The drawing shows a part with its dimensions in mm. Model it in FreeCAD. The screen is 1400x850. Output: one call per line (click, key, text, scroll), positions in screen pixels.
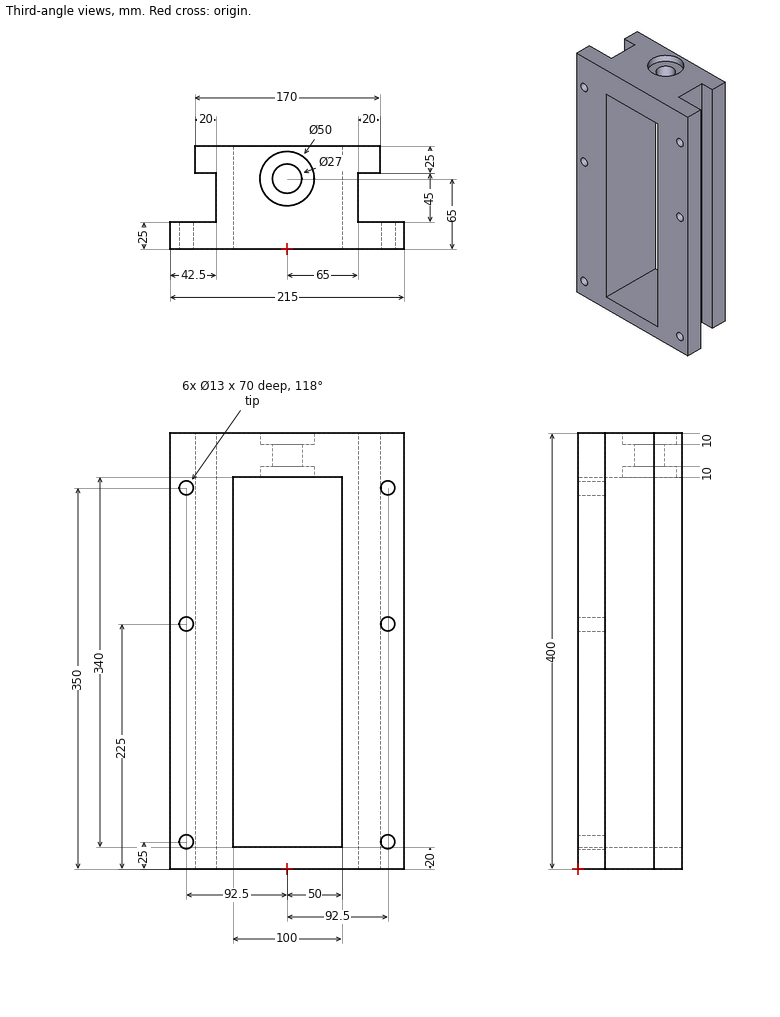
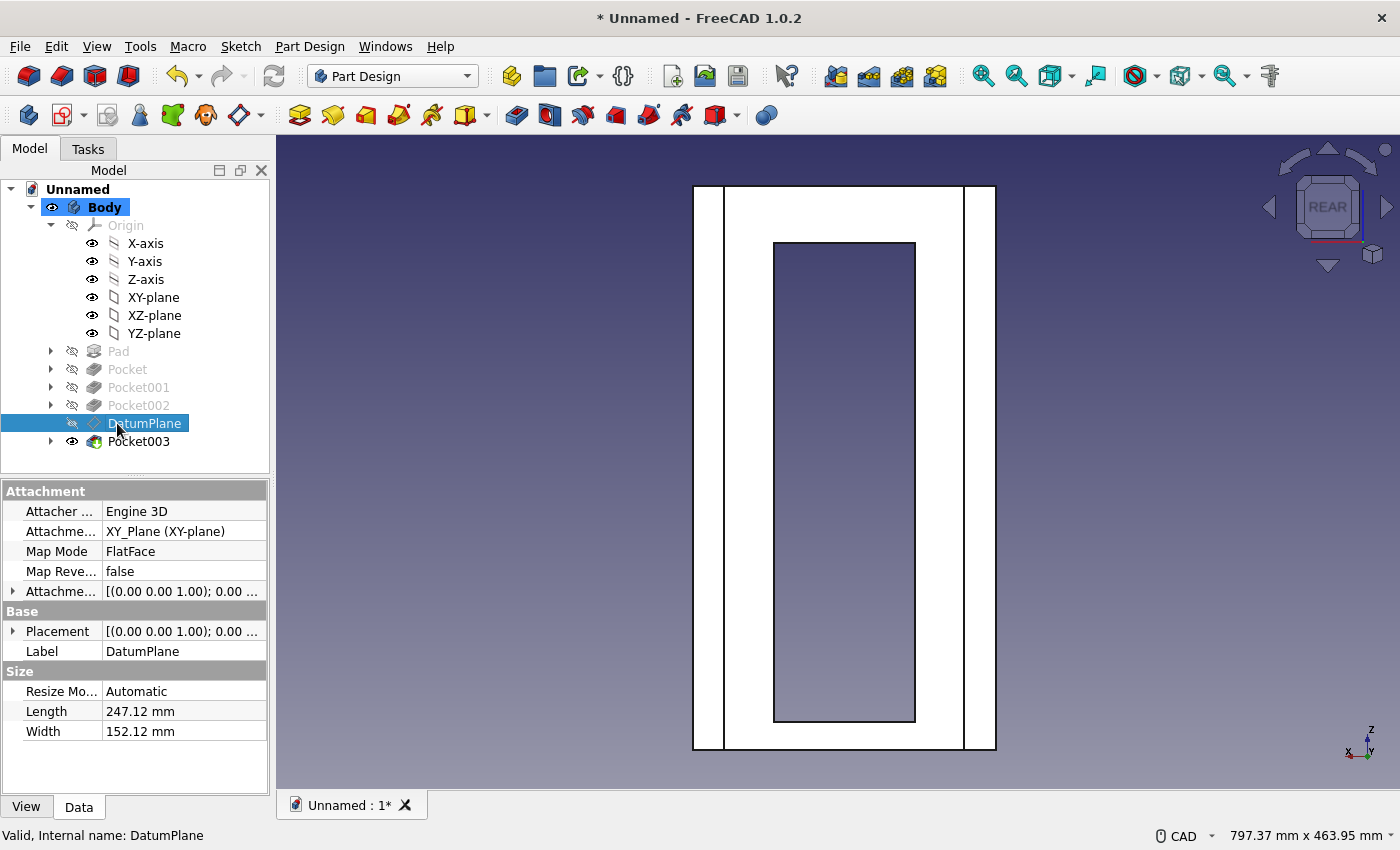
click(714, 226)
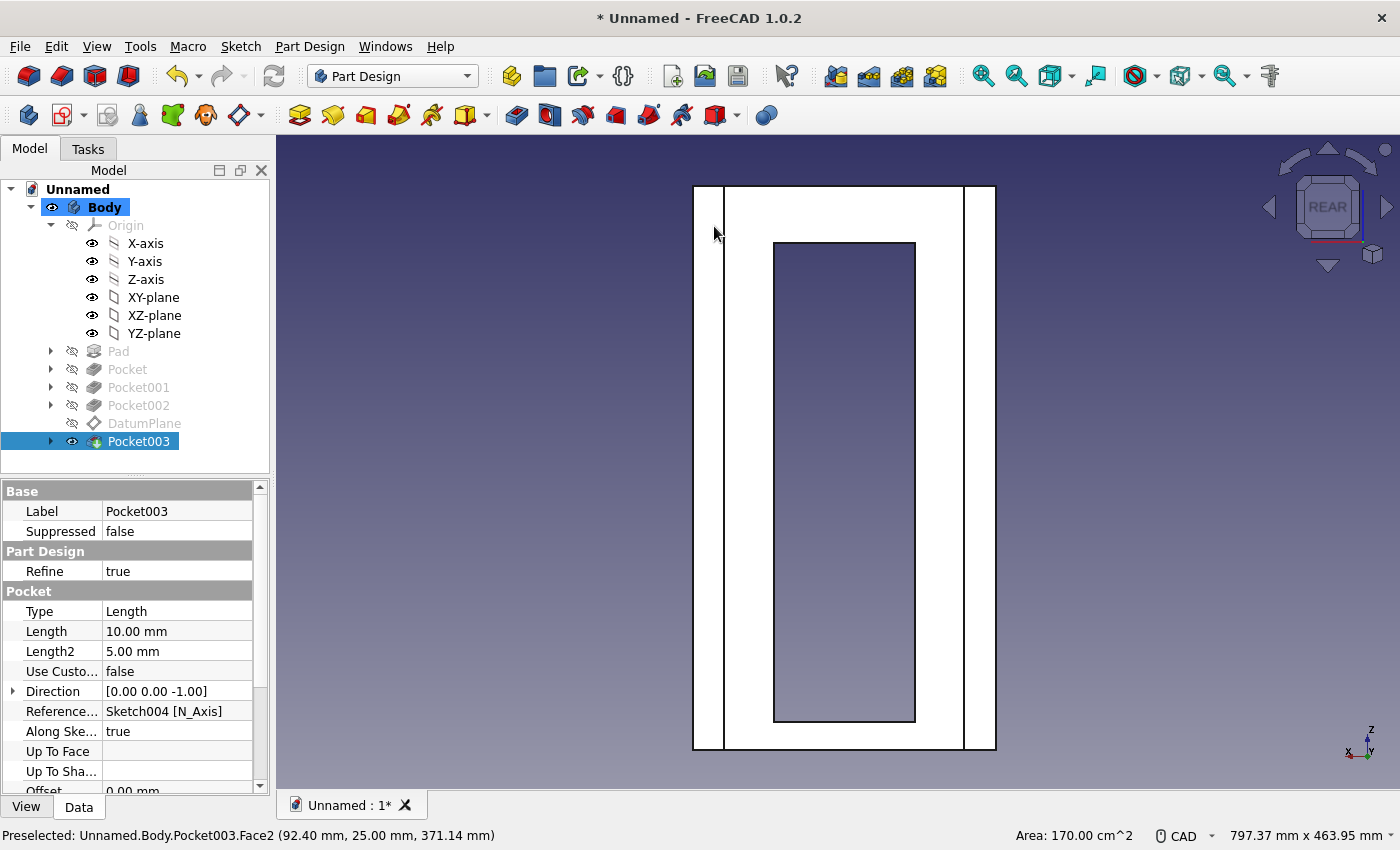
click(62, 116)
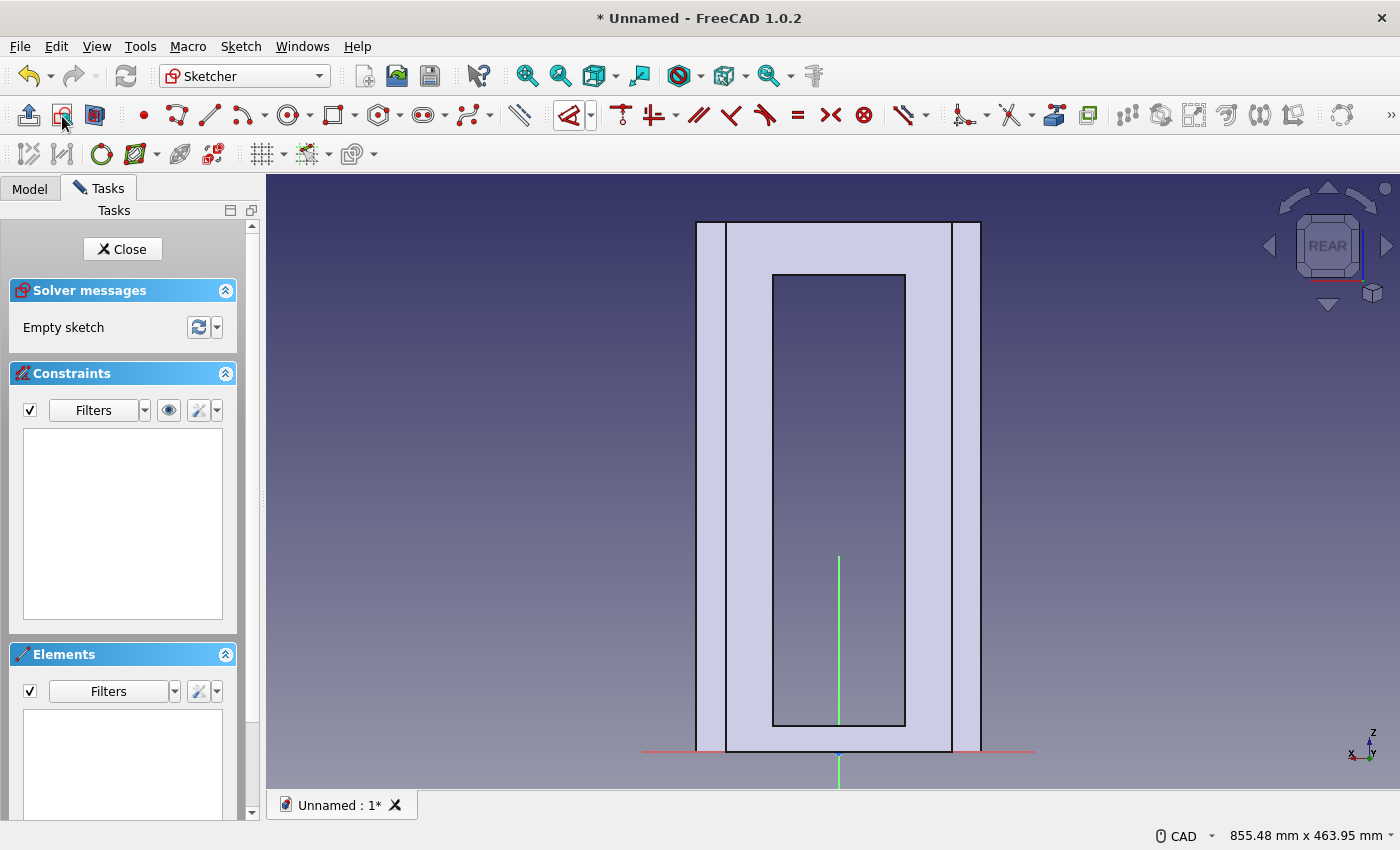
scroll(429, 325, down, 1)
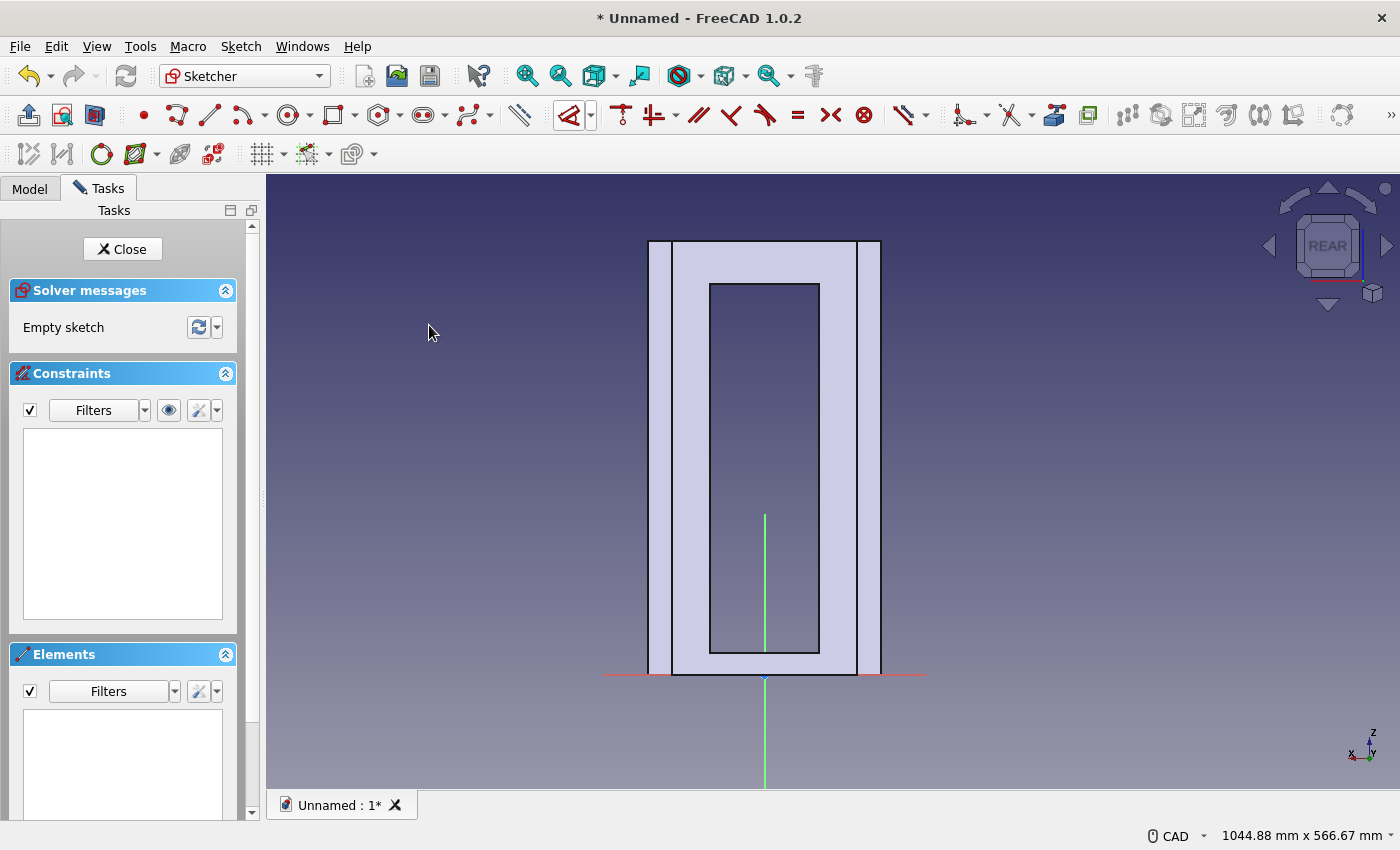
click(288, 116)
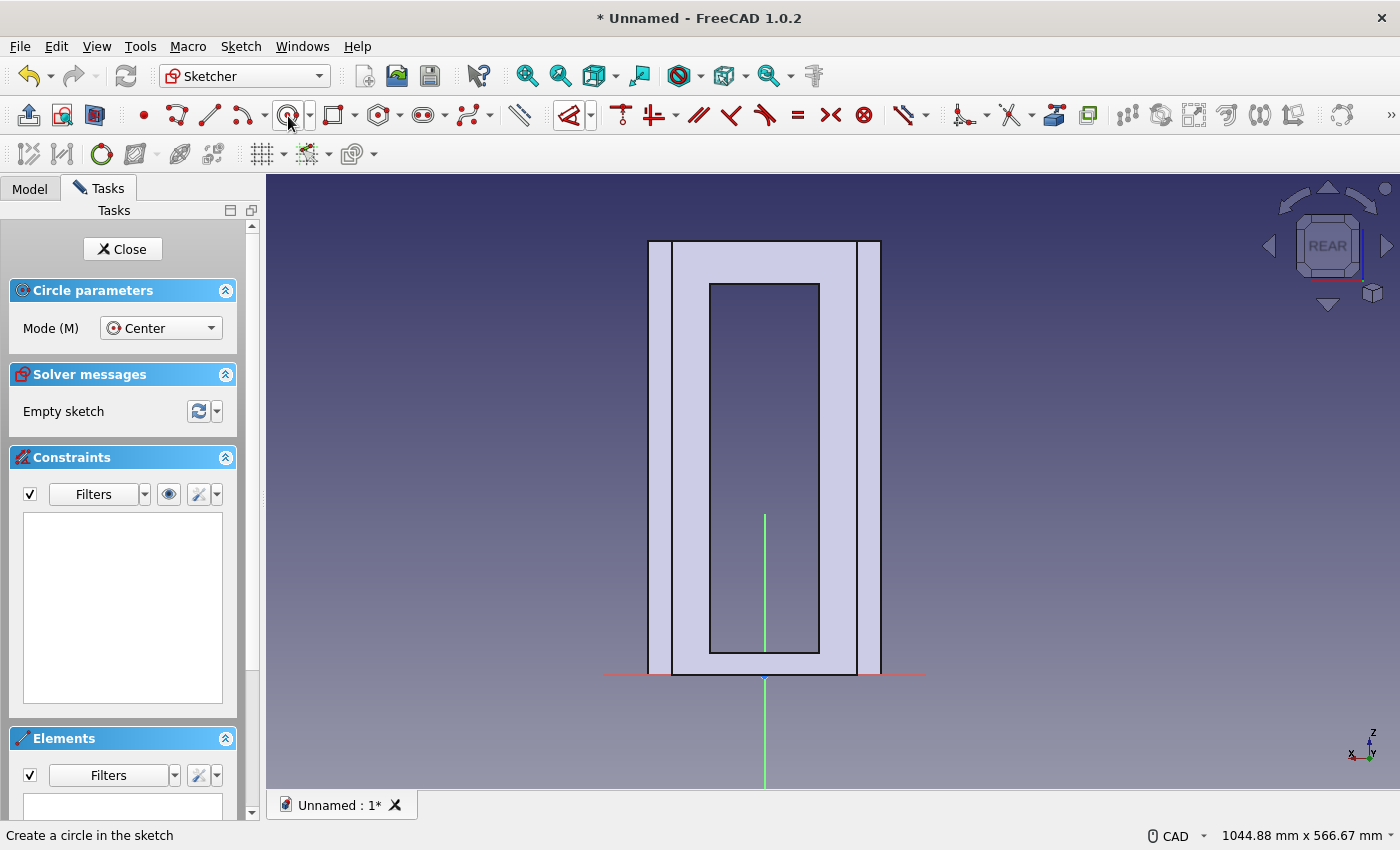
scroll(865, 295, up, 6)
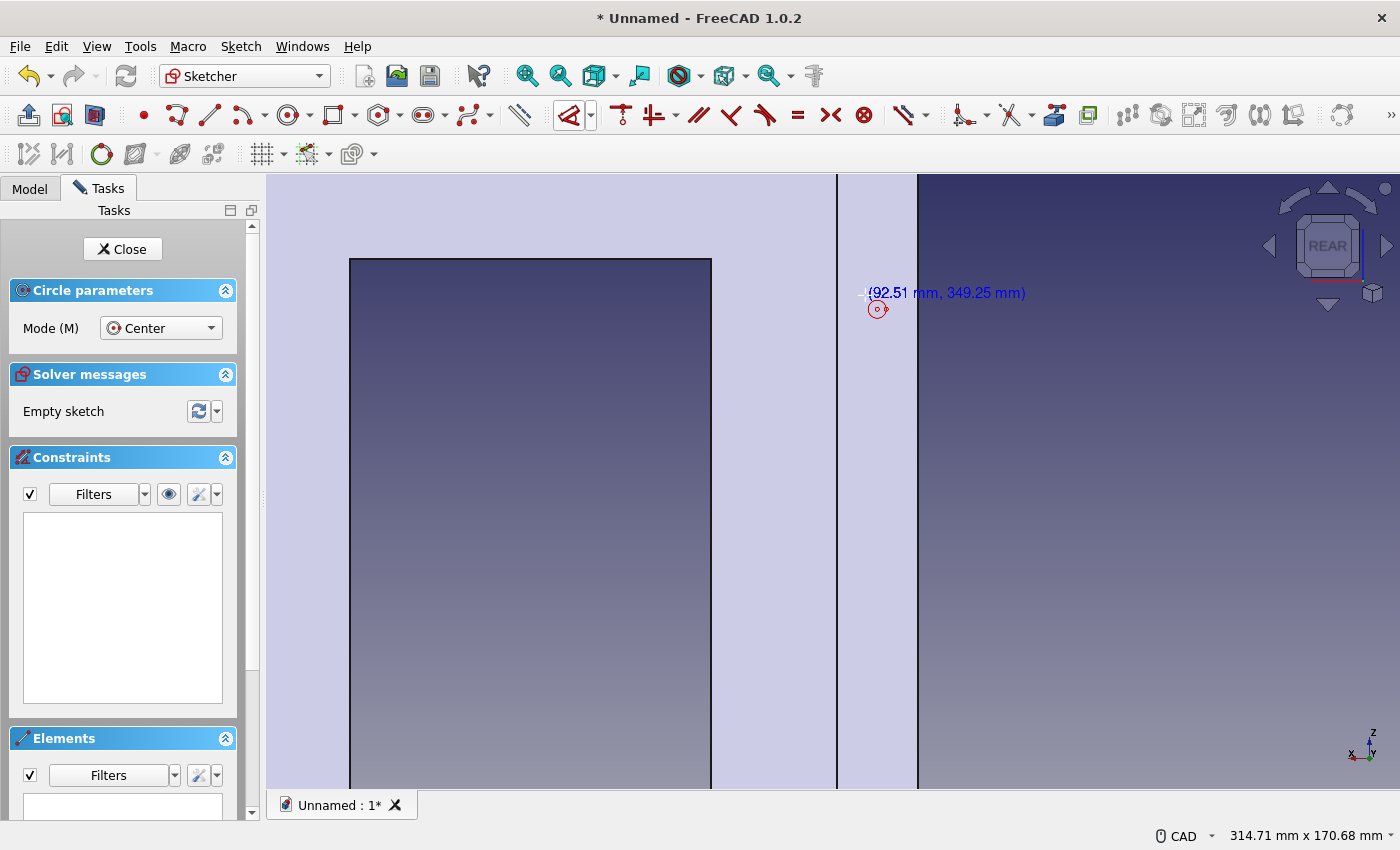
click(864, 295)
move(880, 279)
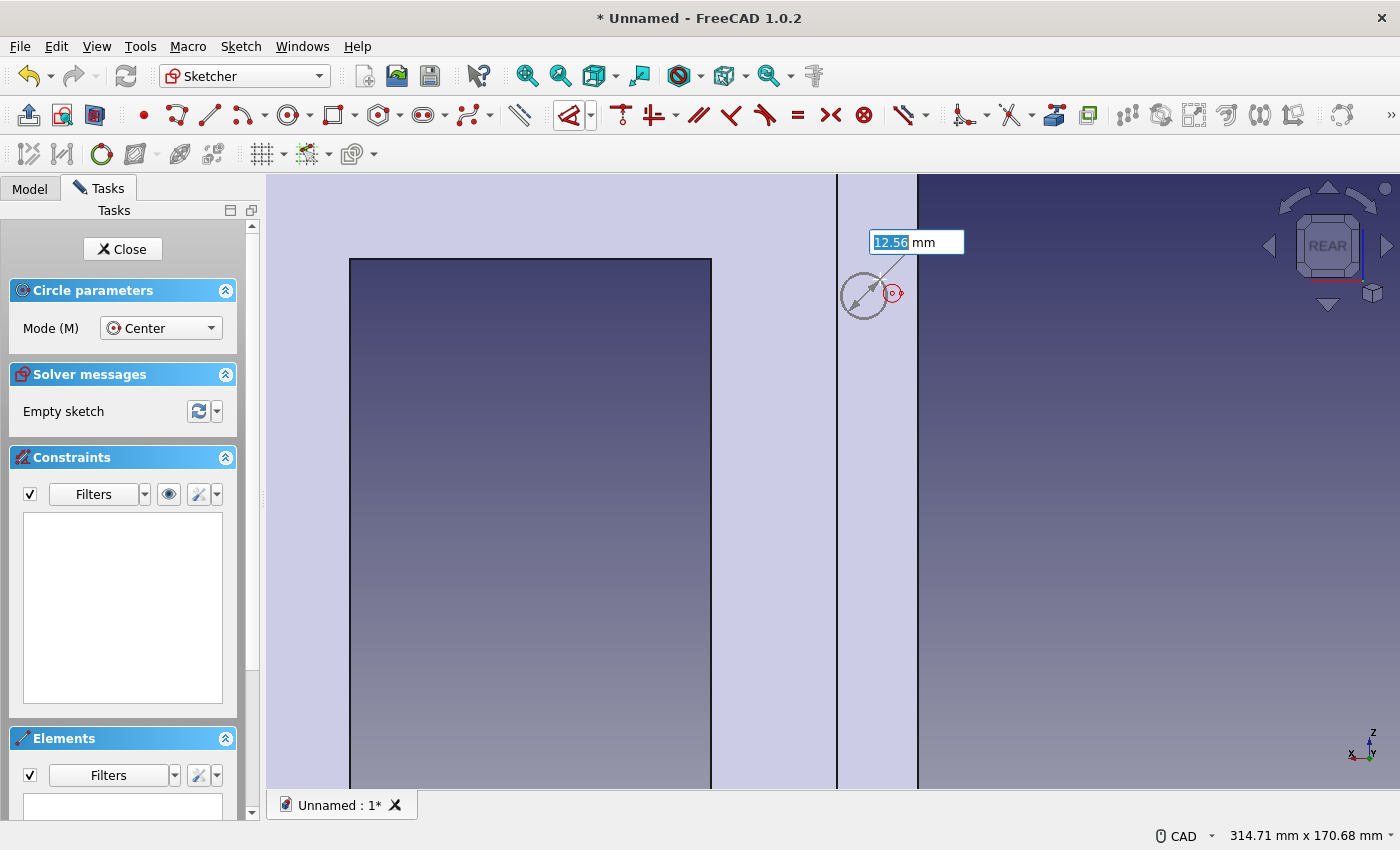
text(13)
key(Return)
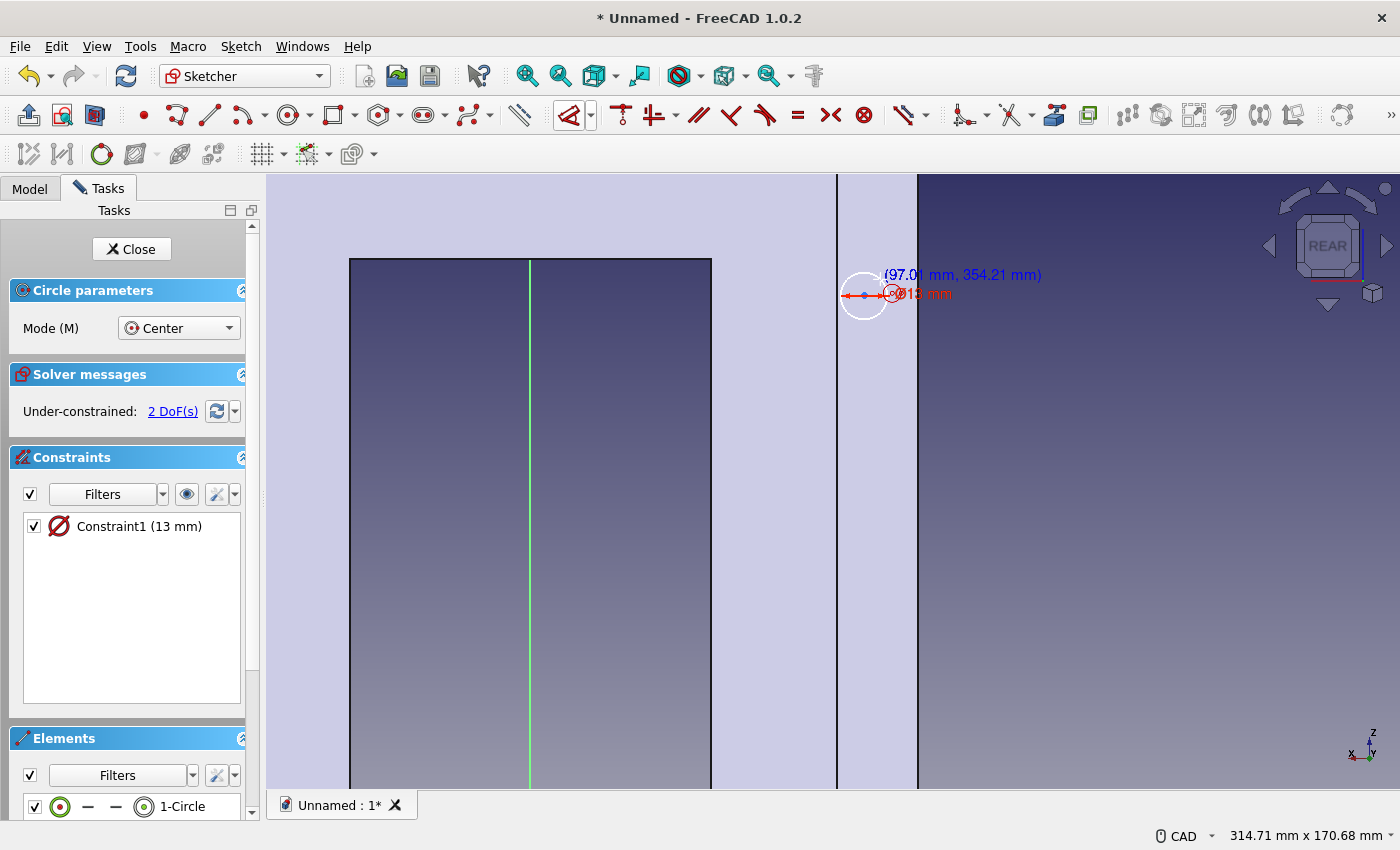
scroll(865, 295, down, 6)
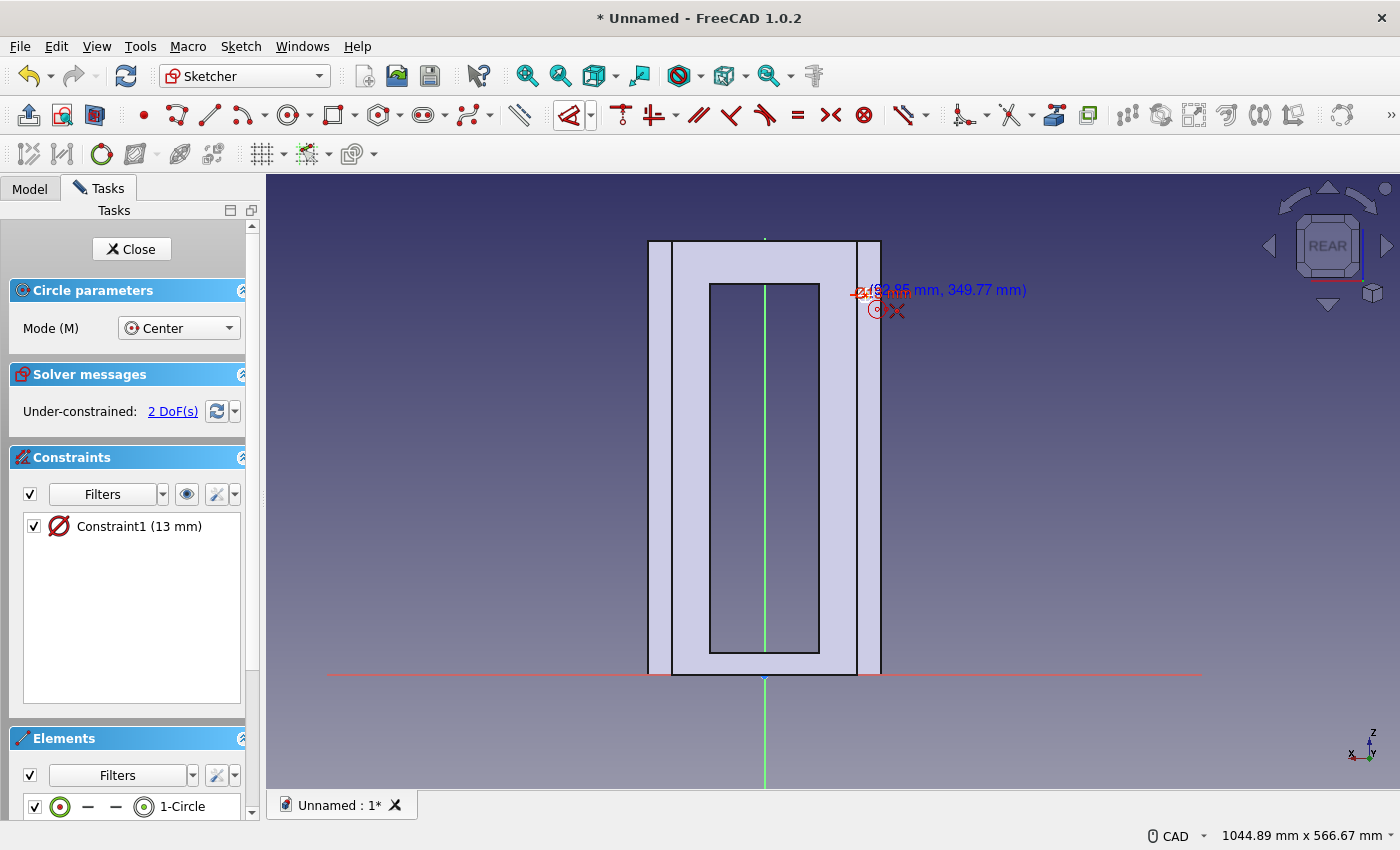
scroll(664, 295, up, 6)